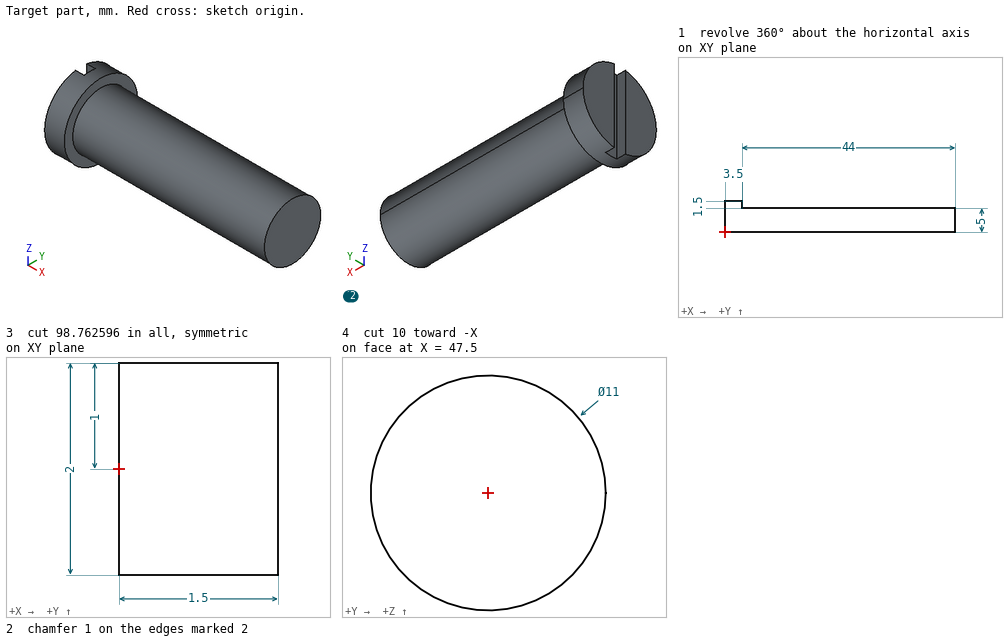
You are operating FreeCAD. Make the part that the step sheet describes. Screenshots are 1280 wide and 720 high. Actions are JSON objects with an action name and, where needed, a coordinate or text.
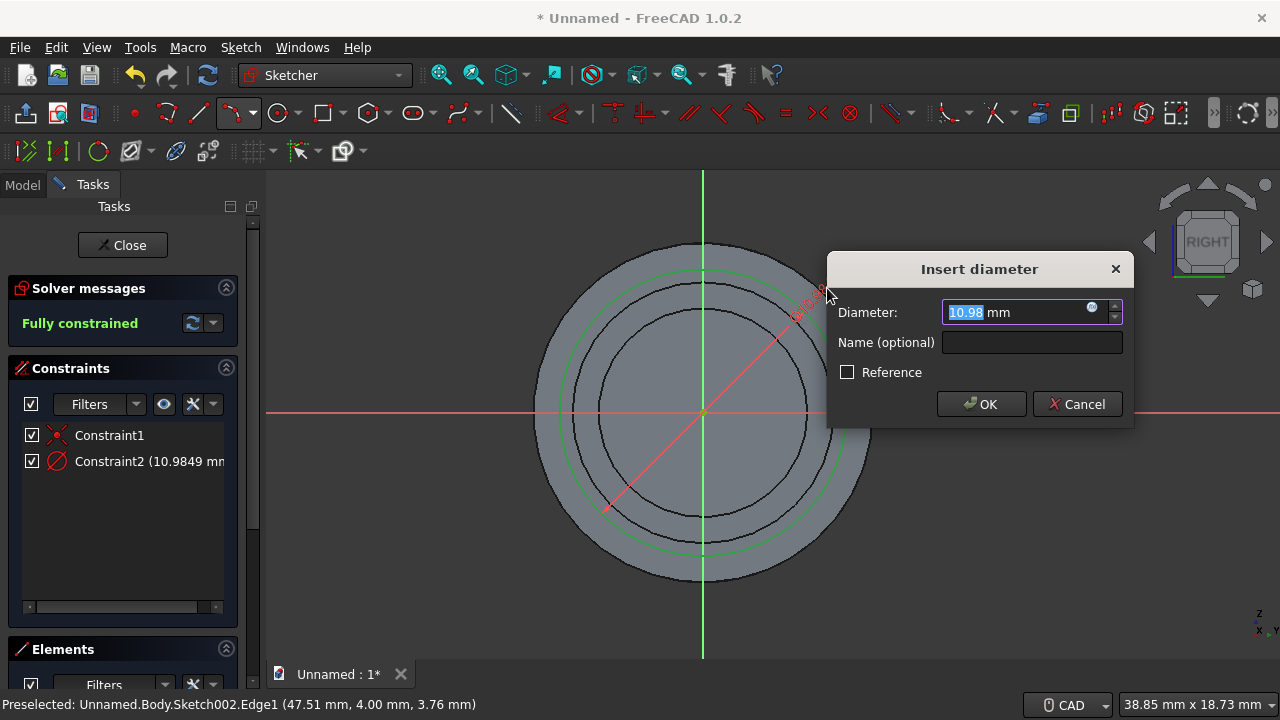
{"action": "type", "text": "11"}
{"action": "key", "text": "Return"}
{"action": "key", "text": "Escape"}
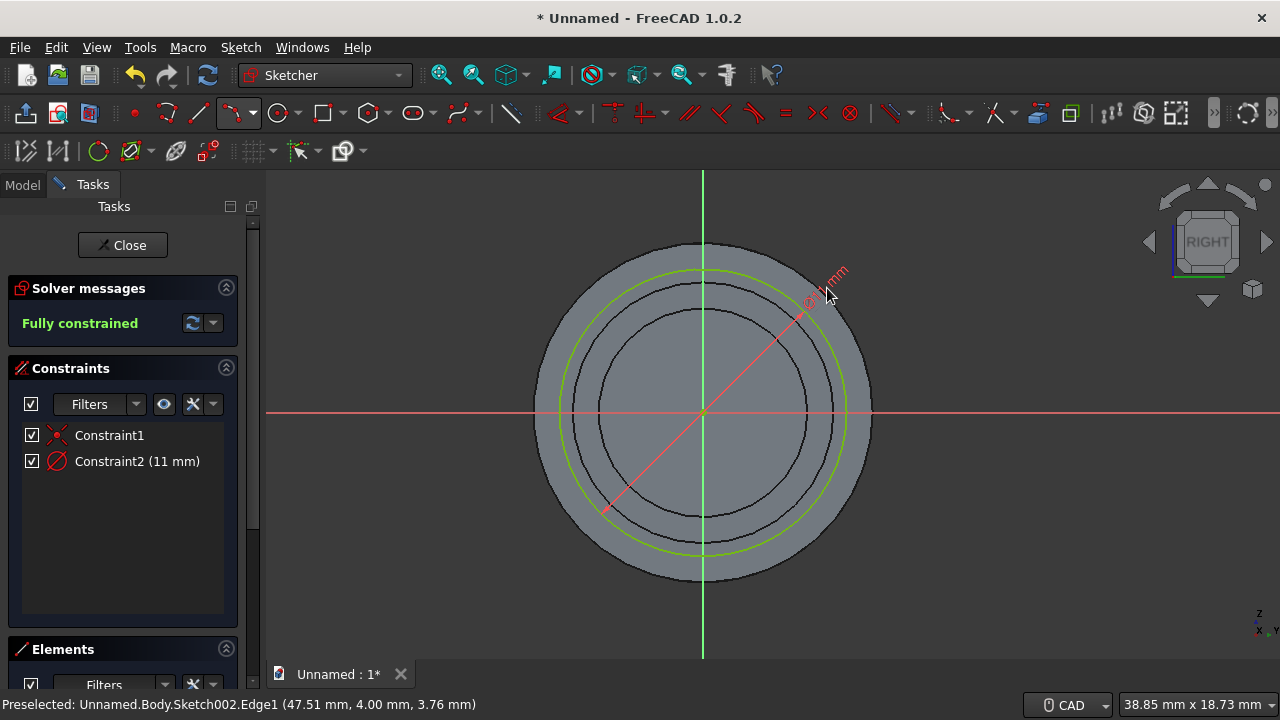
{"action": "left_click", "coordinate": [123, 245]}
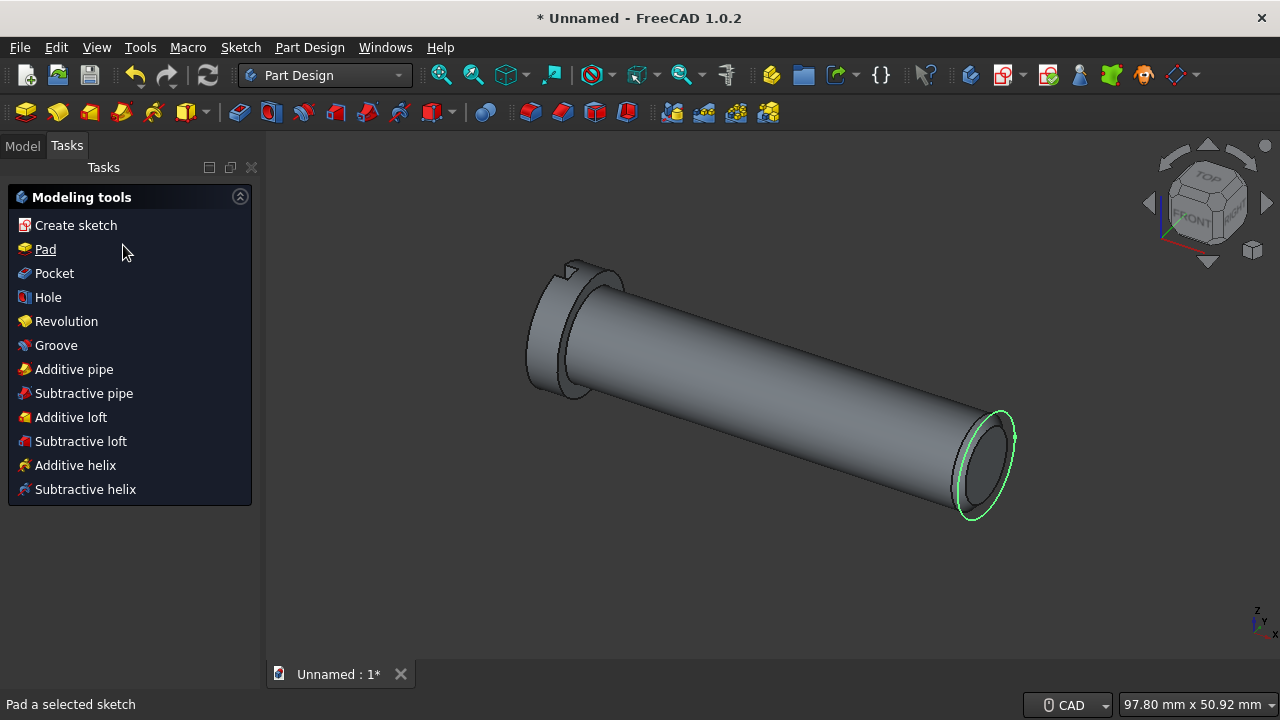
{"action": "left_click", "coordinate": [240, 112]}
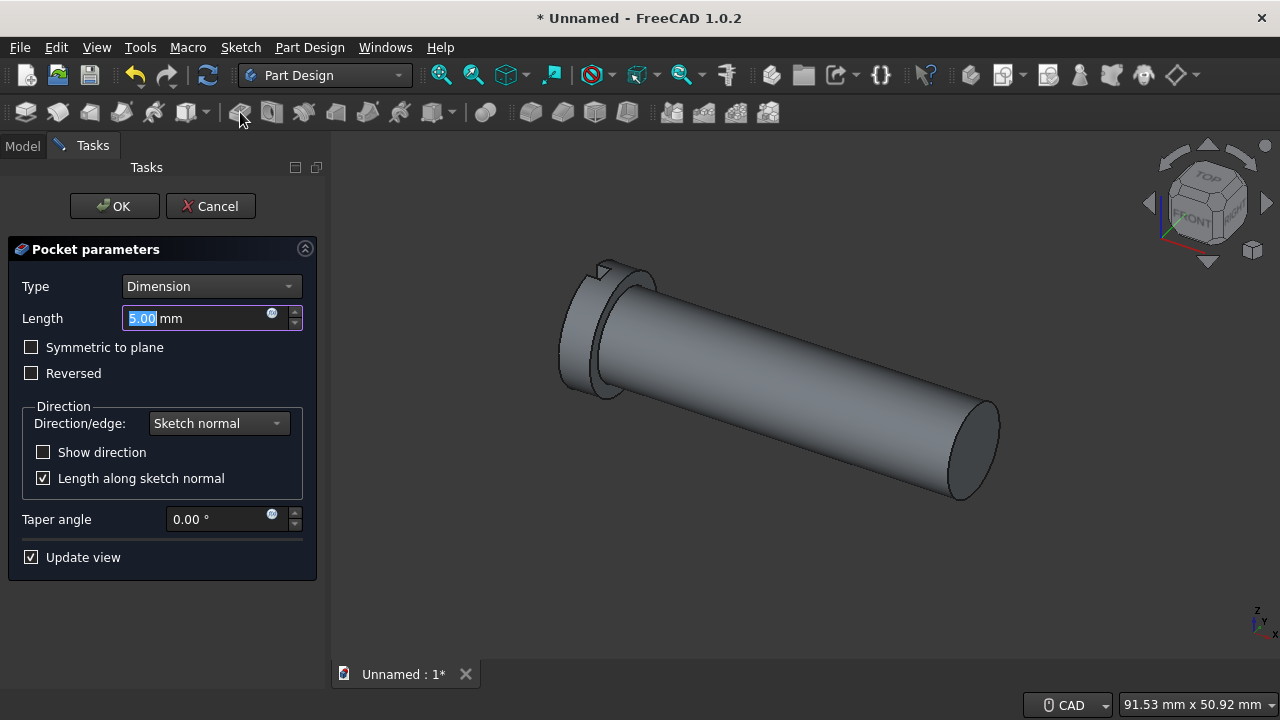
{"action": "type", "text": "10"}
{"action": "key", "text": "Tab"}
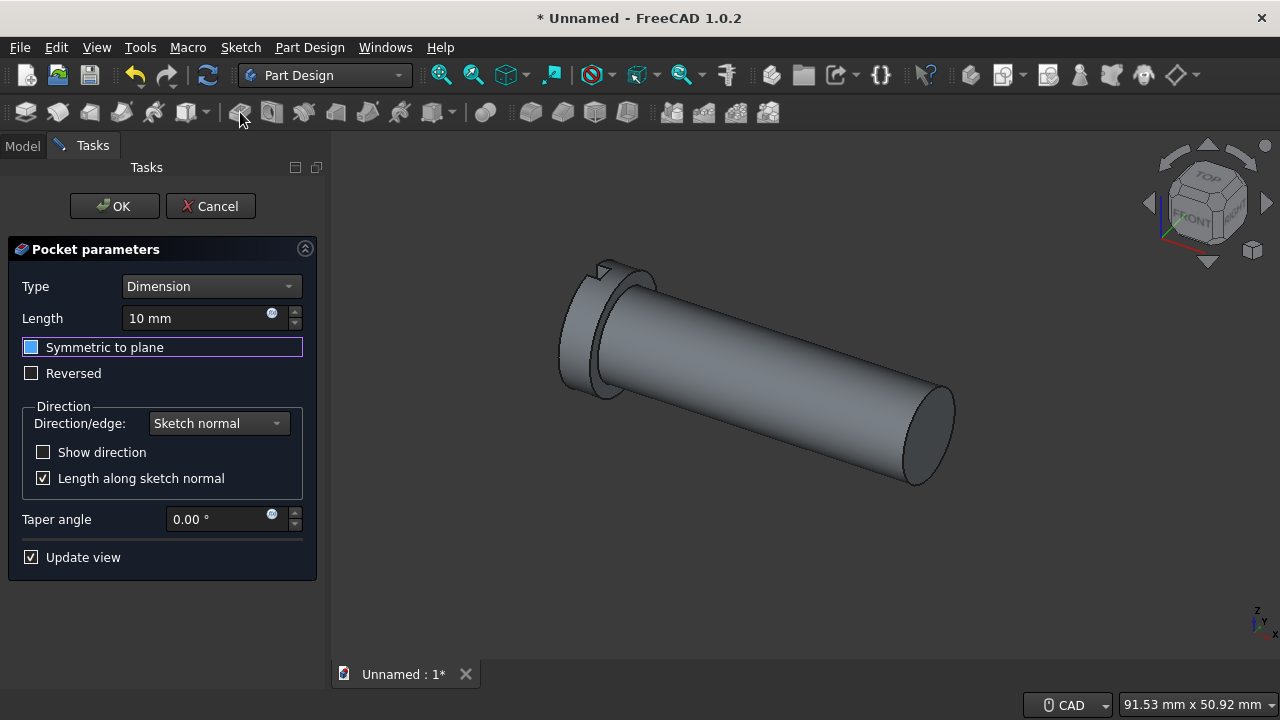
{"action": "left_click", "coordinate": [115, 206]}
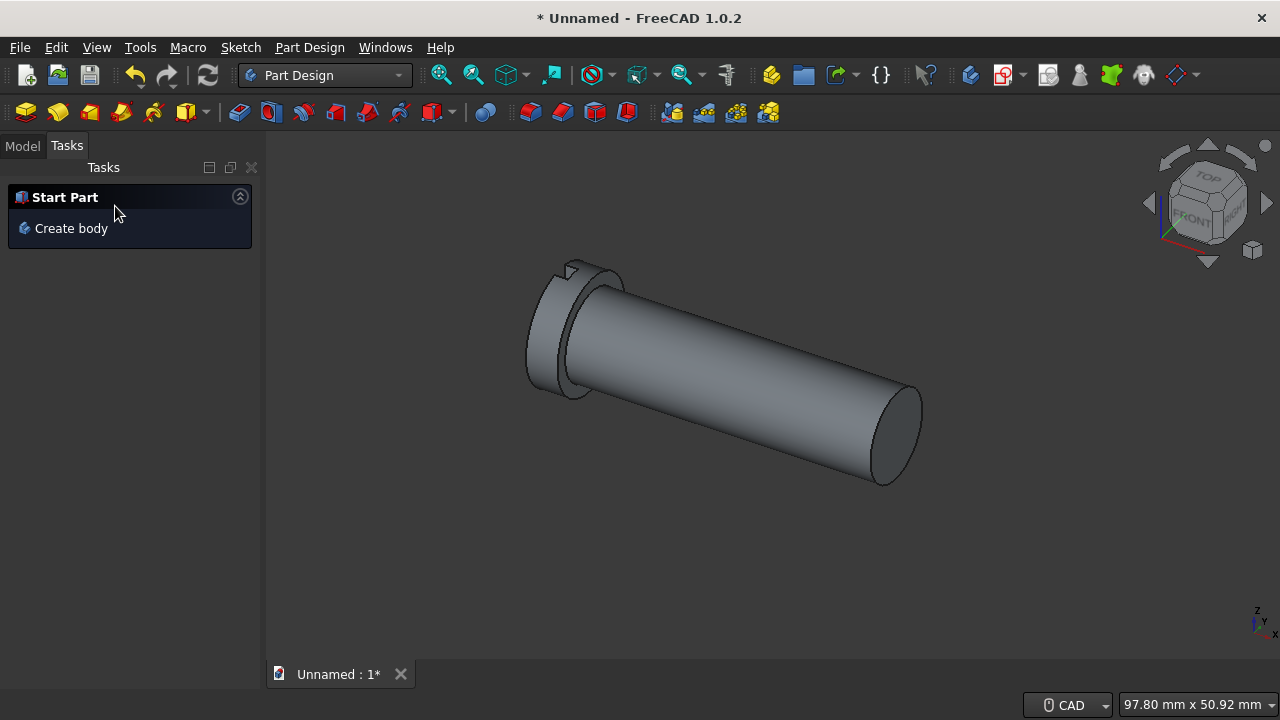
{"action": "key", "text": "0"}